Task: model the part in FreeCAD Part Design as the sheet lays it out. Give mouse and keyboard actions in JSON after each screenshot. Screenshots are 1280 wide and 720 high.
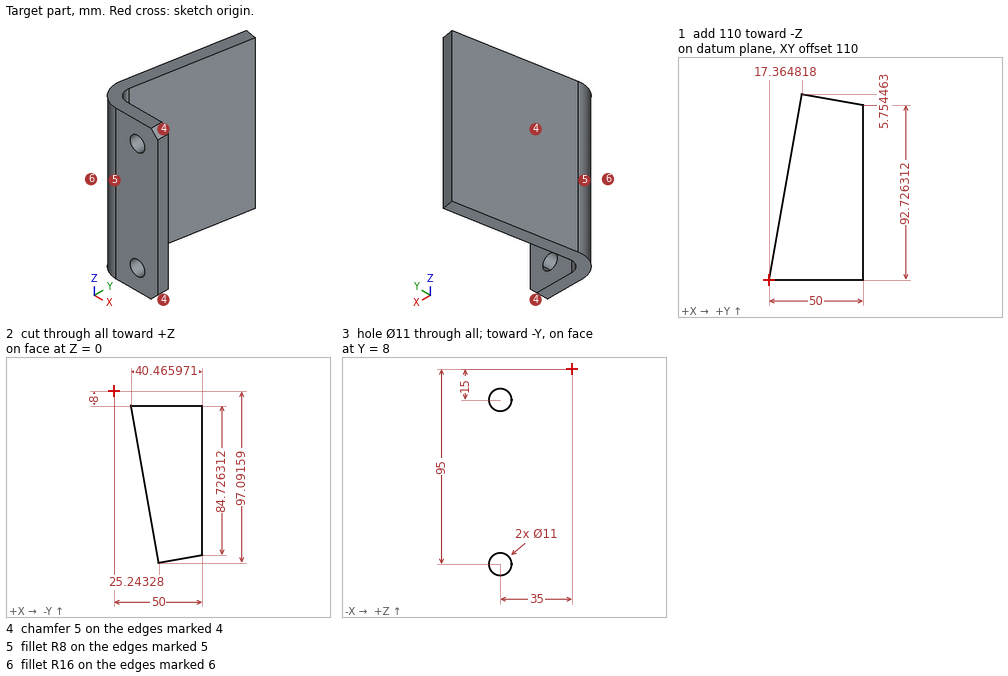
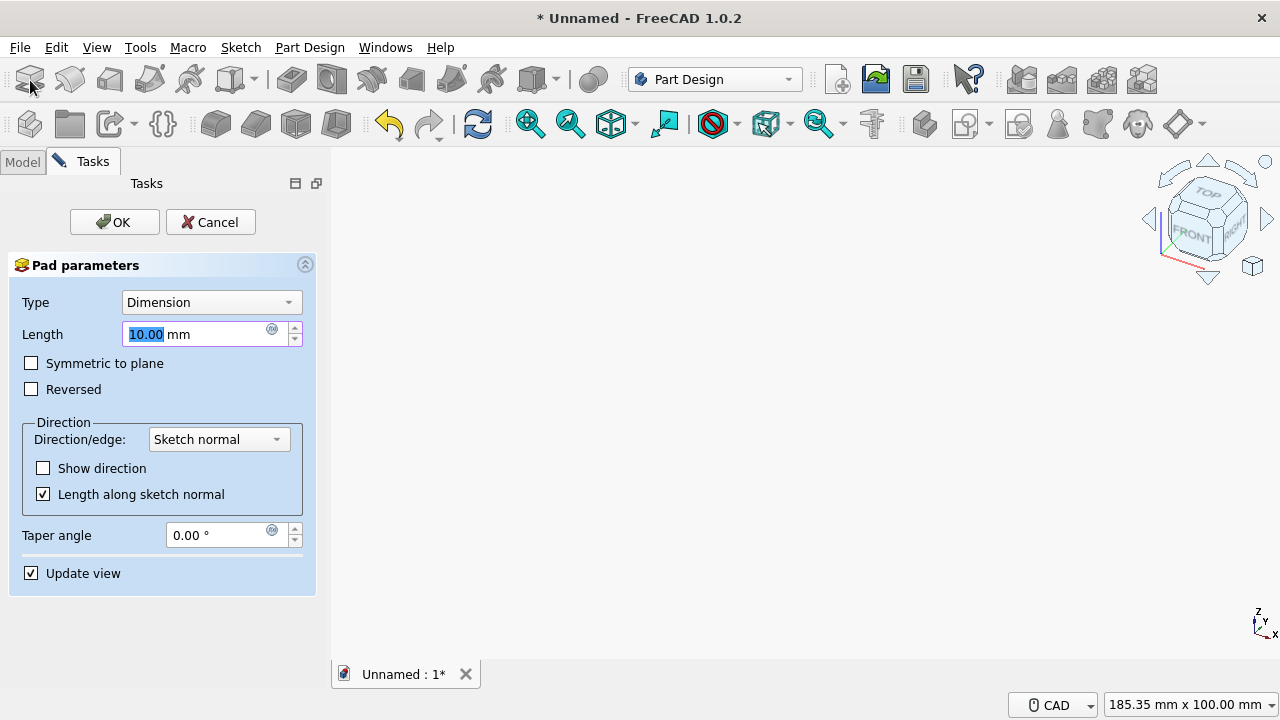
{"action": "type", "text": "110"}
{"action": "key", "text": "Tab"}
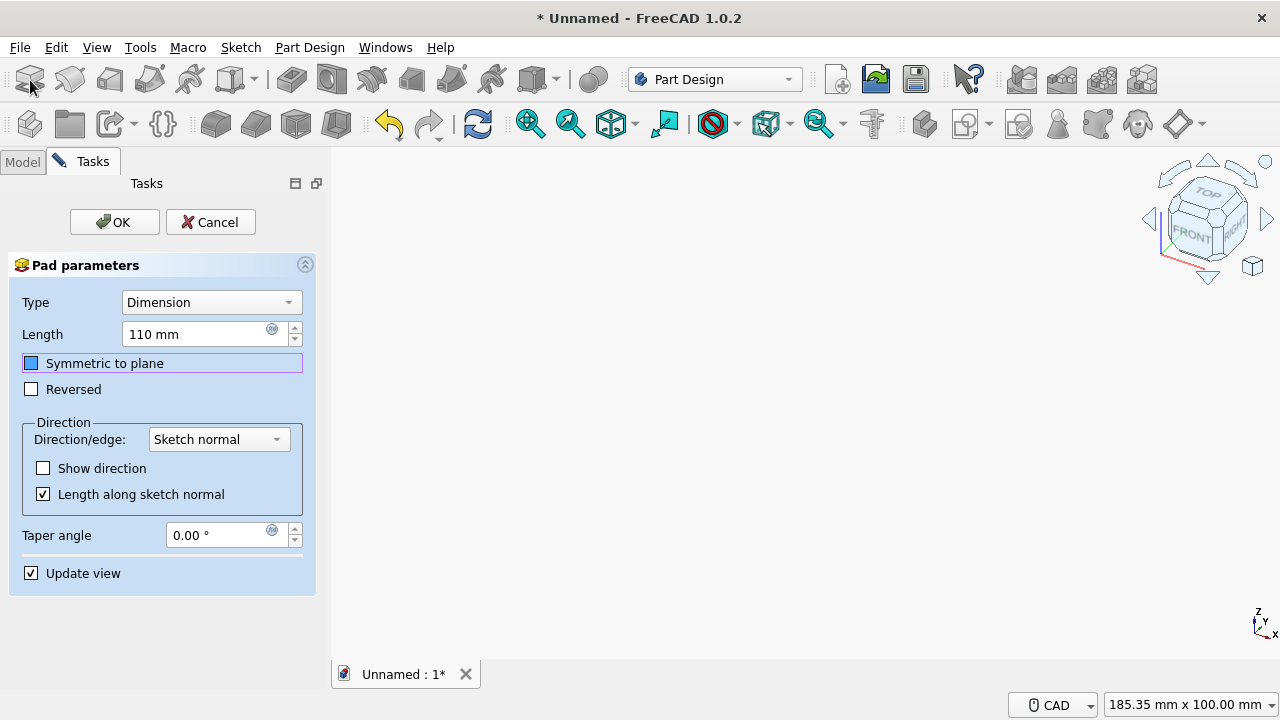
{"action": "left_click", "coordinate": [30, 389]}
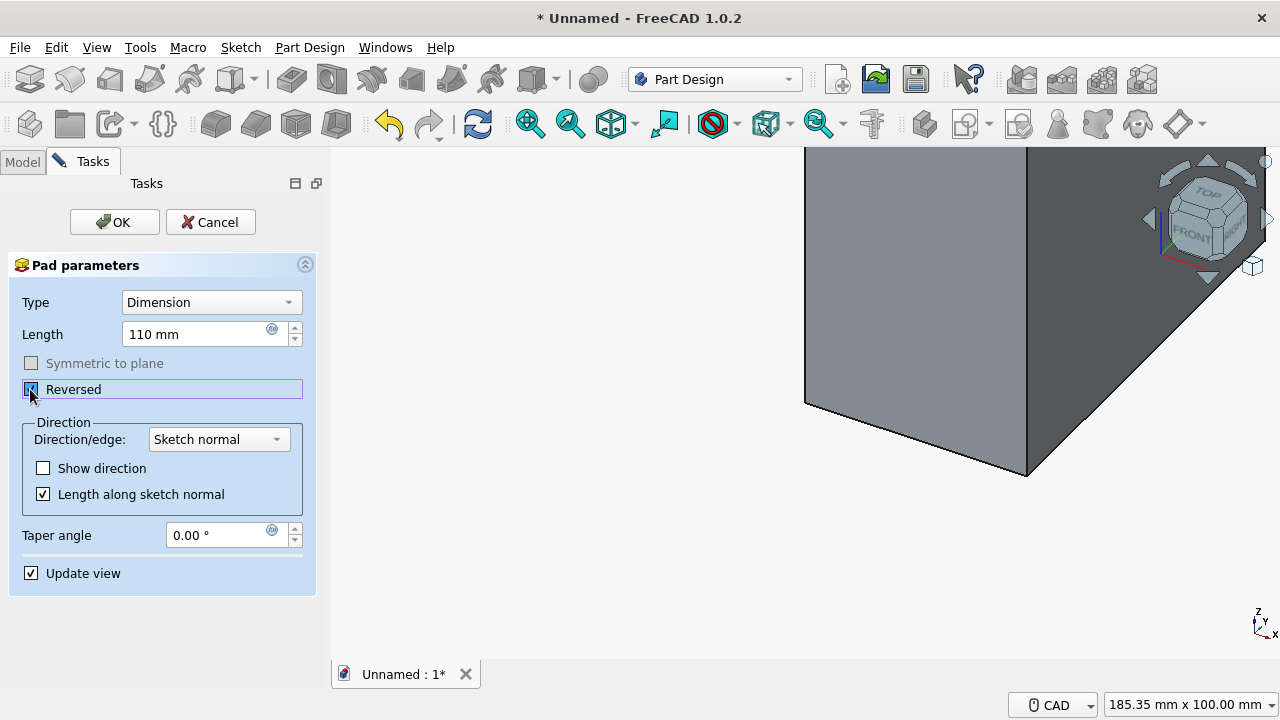
{"action": "left_click", "coordinate": [115, 222]}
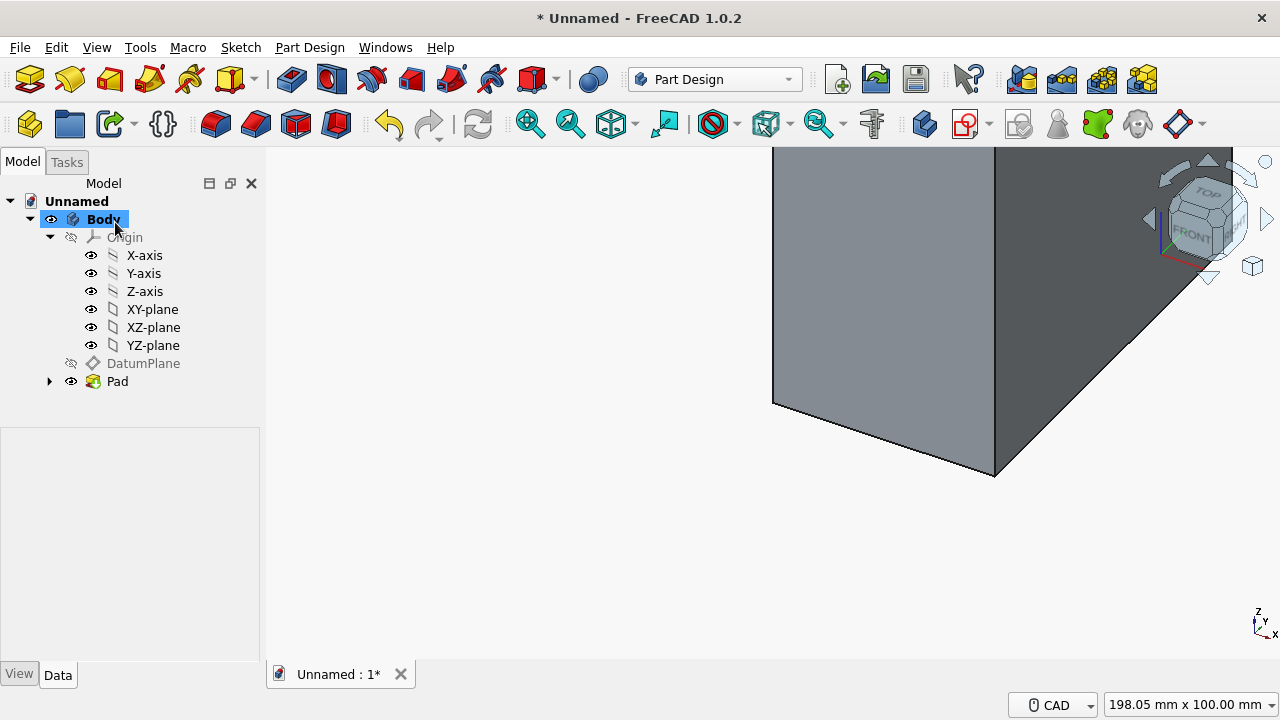
{"action": "key", "text": "v f"}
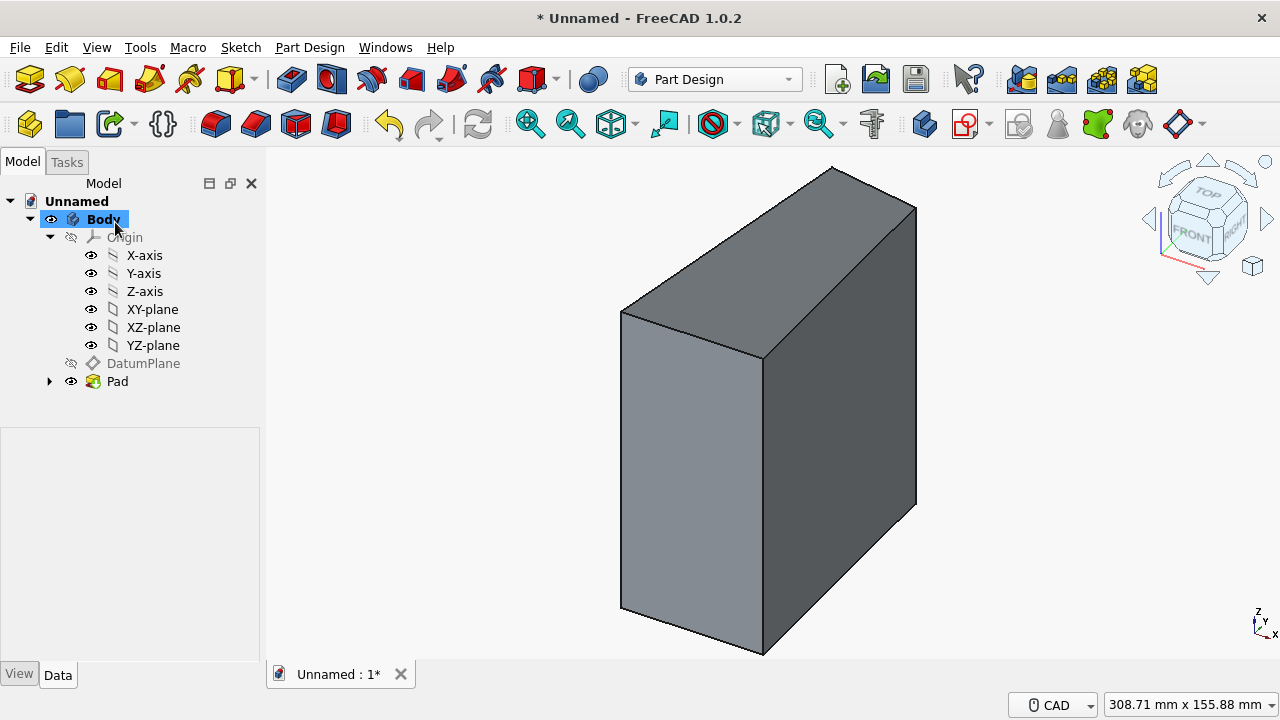
{"action": "key", "text": "5"}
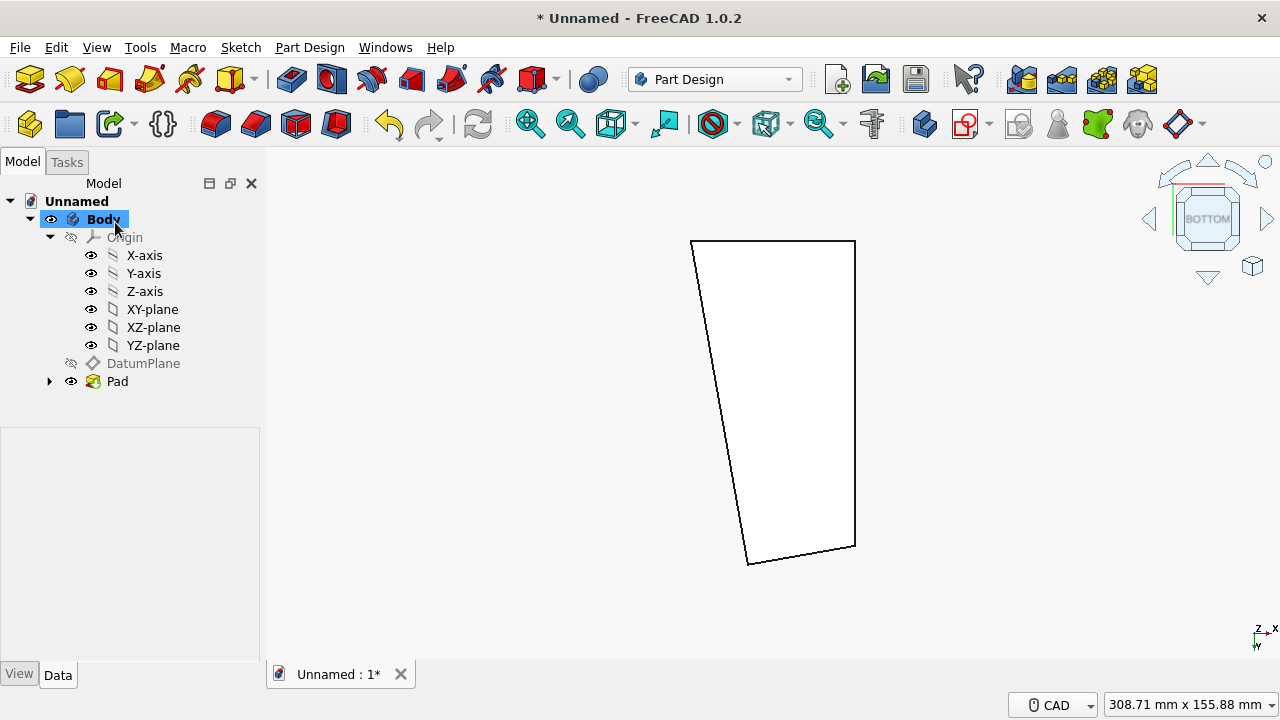
{"action": "left_click", "coordinate": [773, 310]}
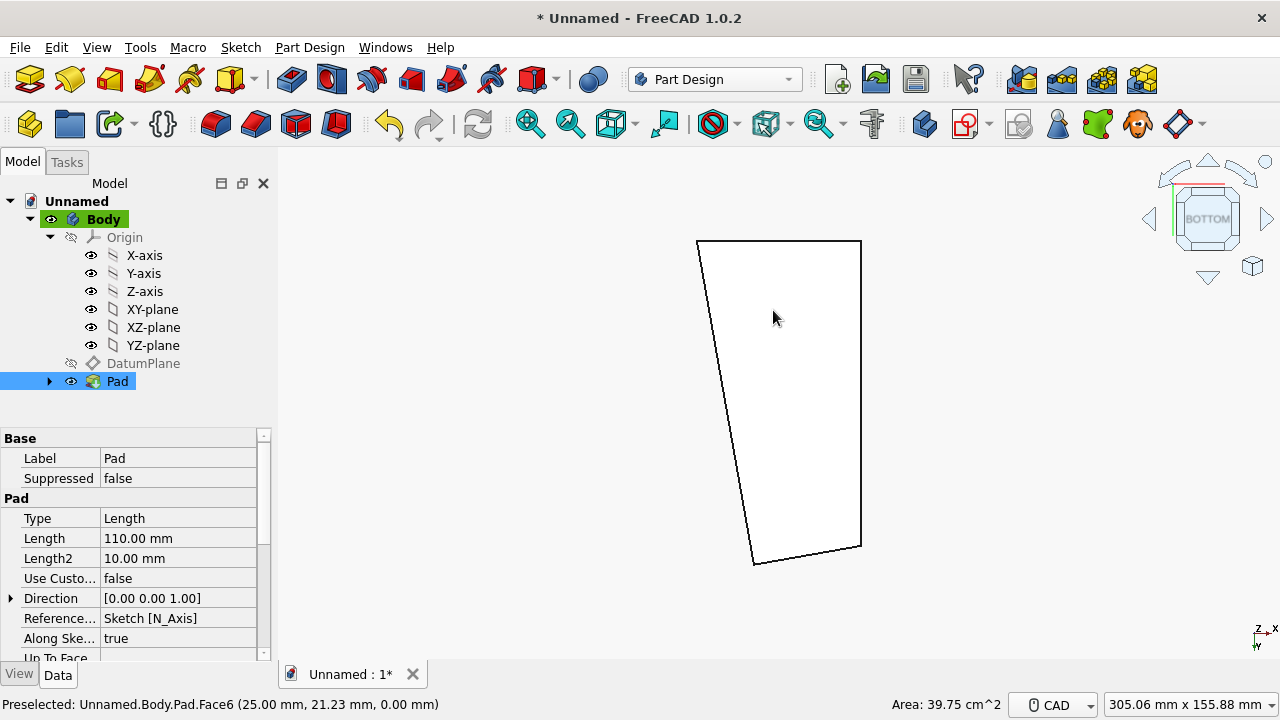
{"action": "left_click", "coordinate": [966, 124]}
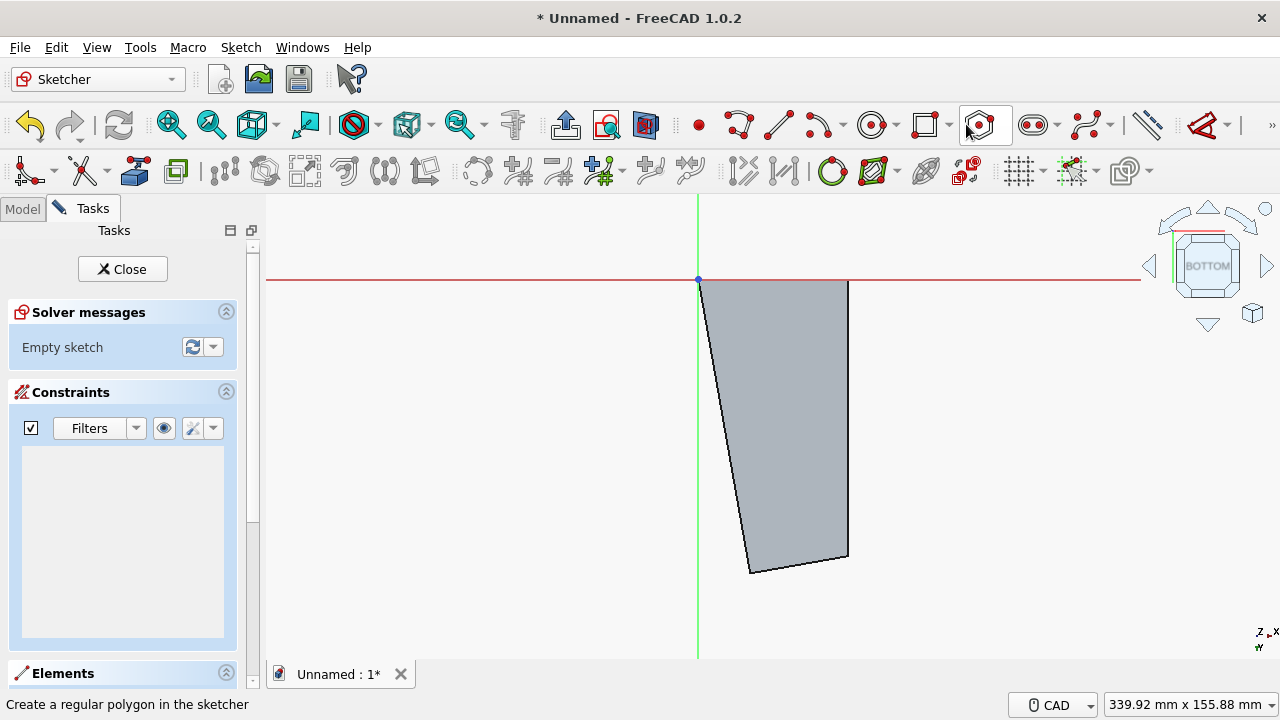
{"action": "left_click", "coordinate": [740, 126]}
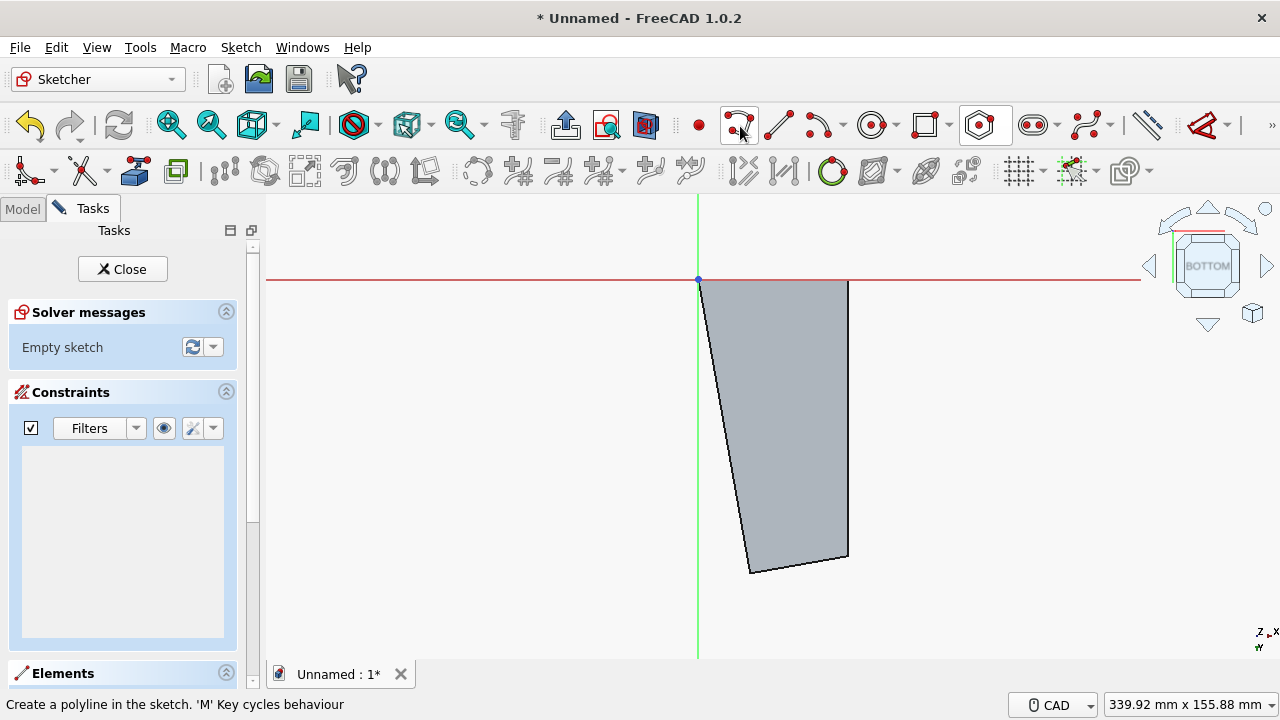
{"action": "left_click", "coordinate": [727, 303]}
{"action": "left_click", "coordinate": [774, 569]}
{"action": "left_click", "coordinate": [848, 556]}
{"action": "left_click", "coordinate": [848, 303]}
{"action": "left_click", "coordinate": [727, 304]}
{"action": "key", "text": "Escape"}
{"action": "key", "text": "Escape"}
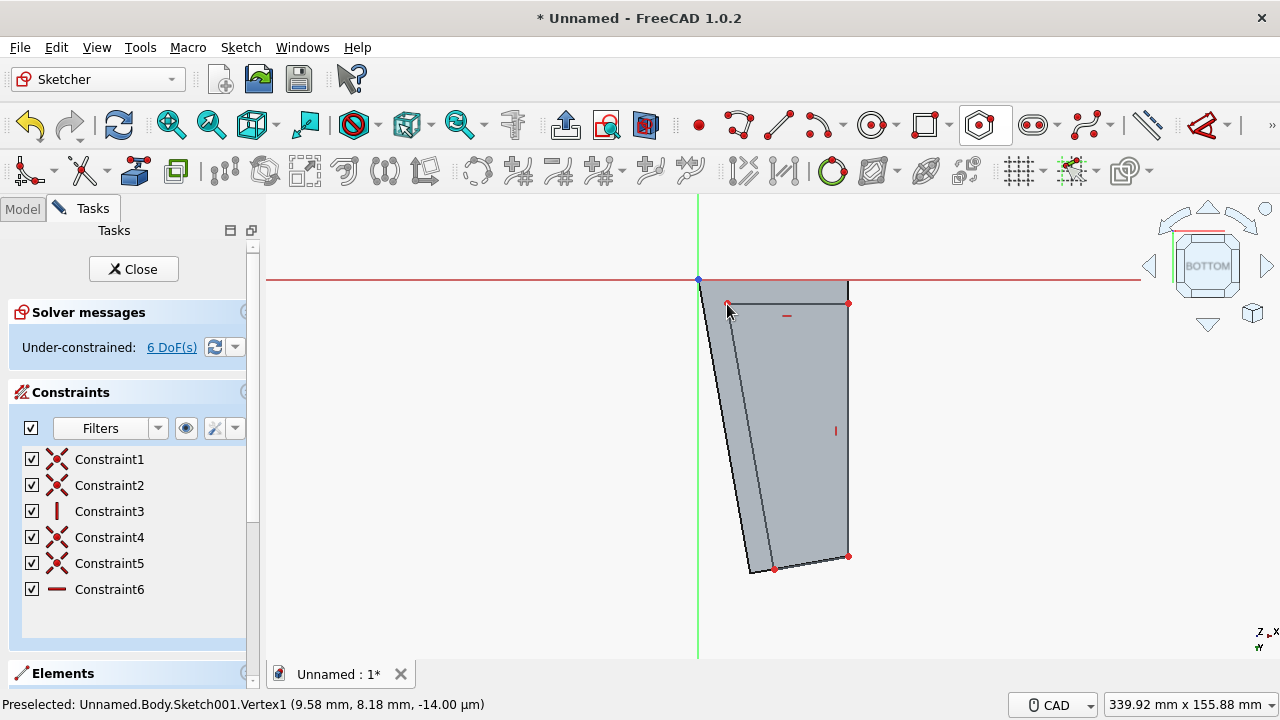
{"action": "scroll", "coordinate": [727, 304], "scroll_direction": "up", "scroll_amount": 3}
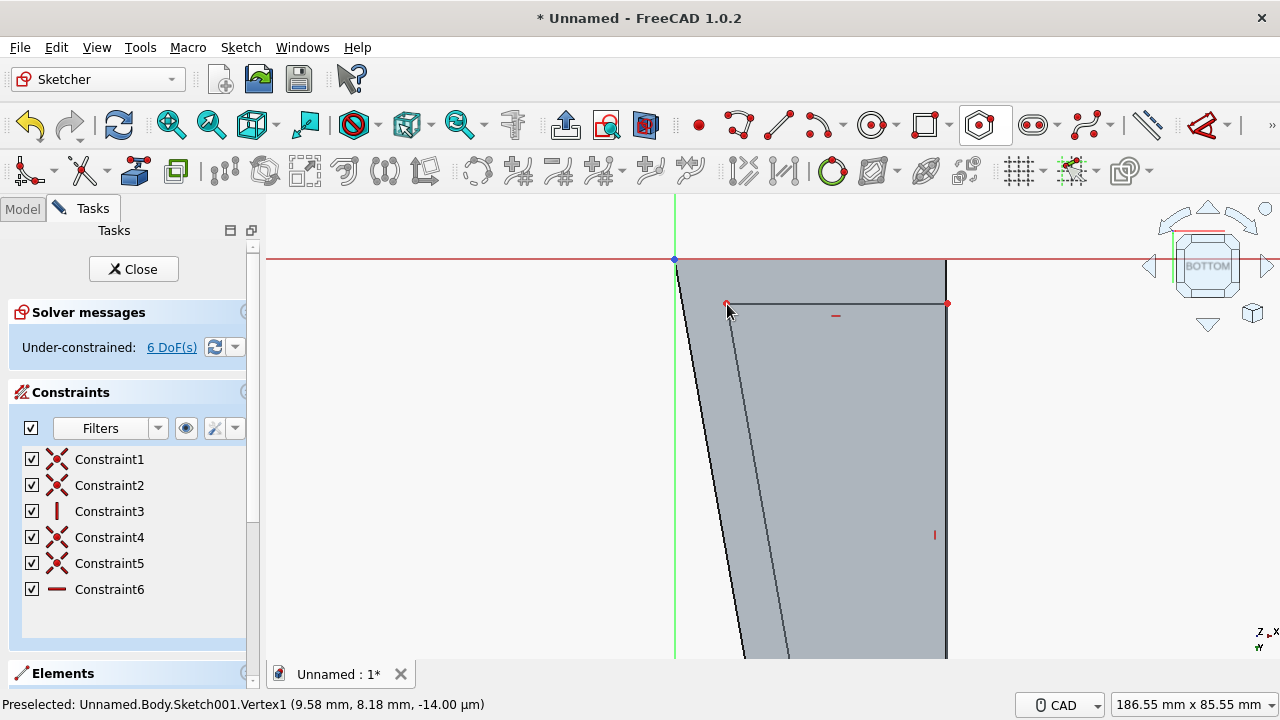
{"action": "left_click", "coordinate": [727, 304]}